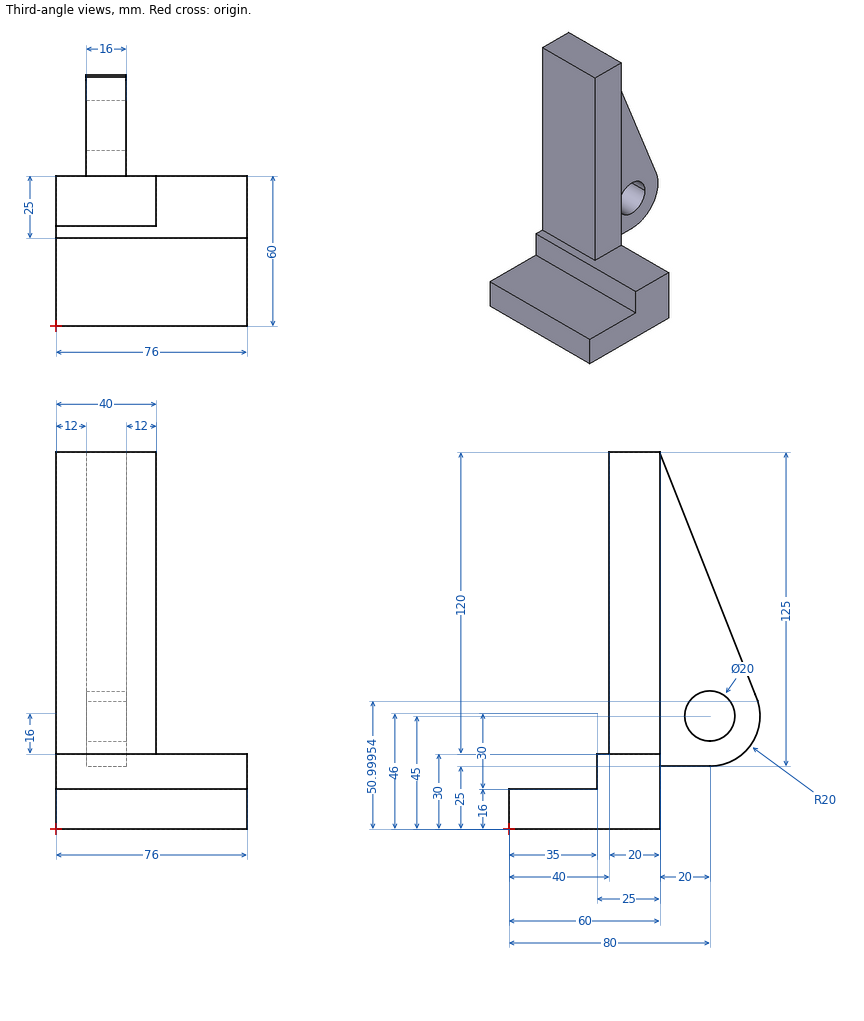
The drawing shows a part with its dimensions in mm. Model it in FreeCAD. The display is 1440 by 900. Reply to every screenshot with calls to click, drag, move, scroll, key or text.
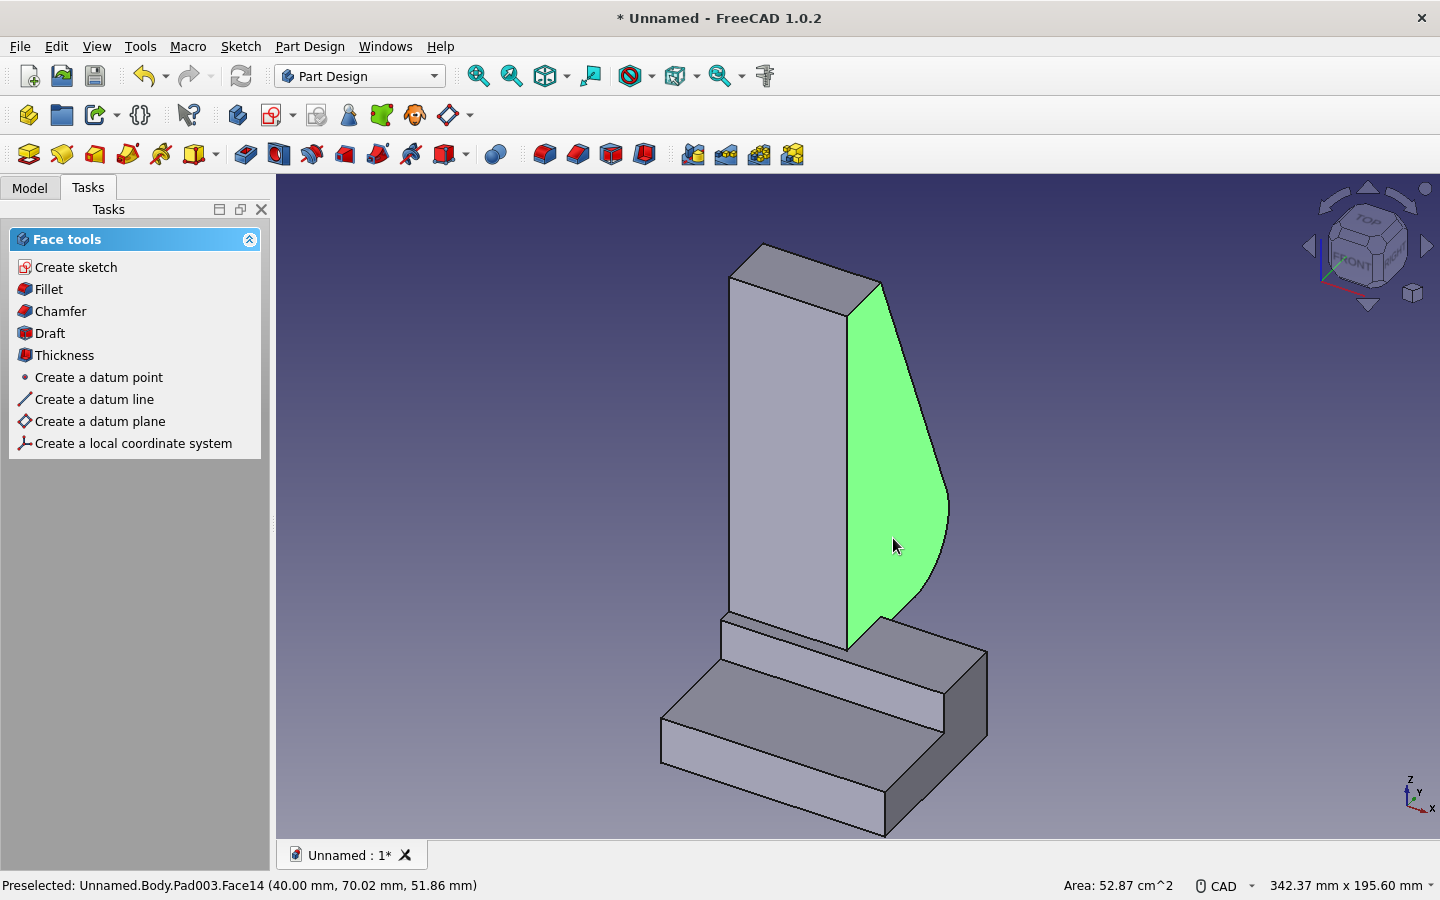
click(270, 116)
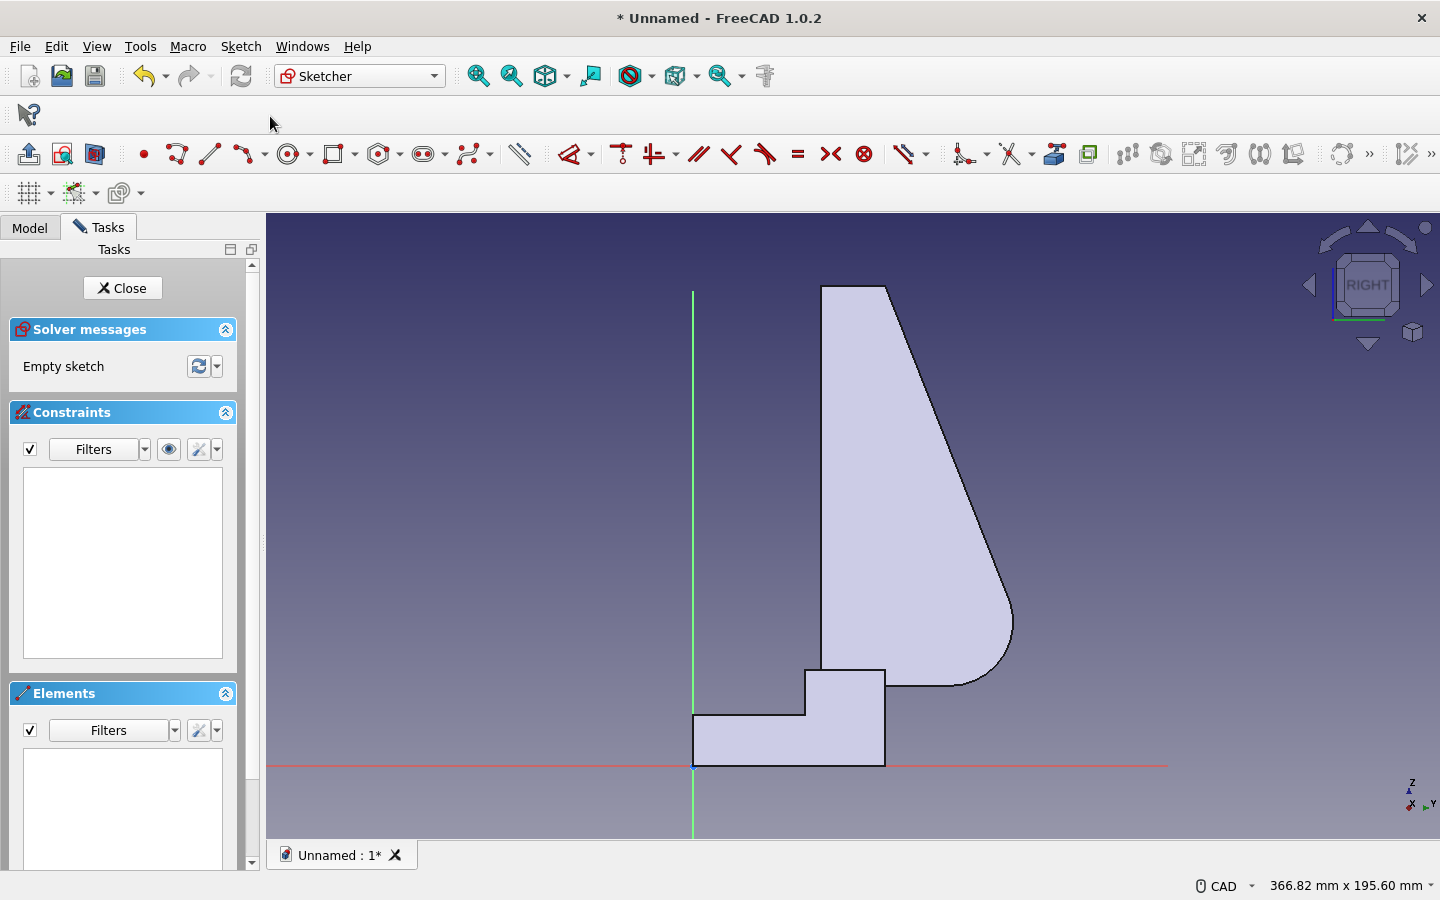
key(g)
key(m)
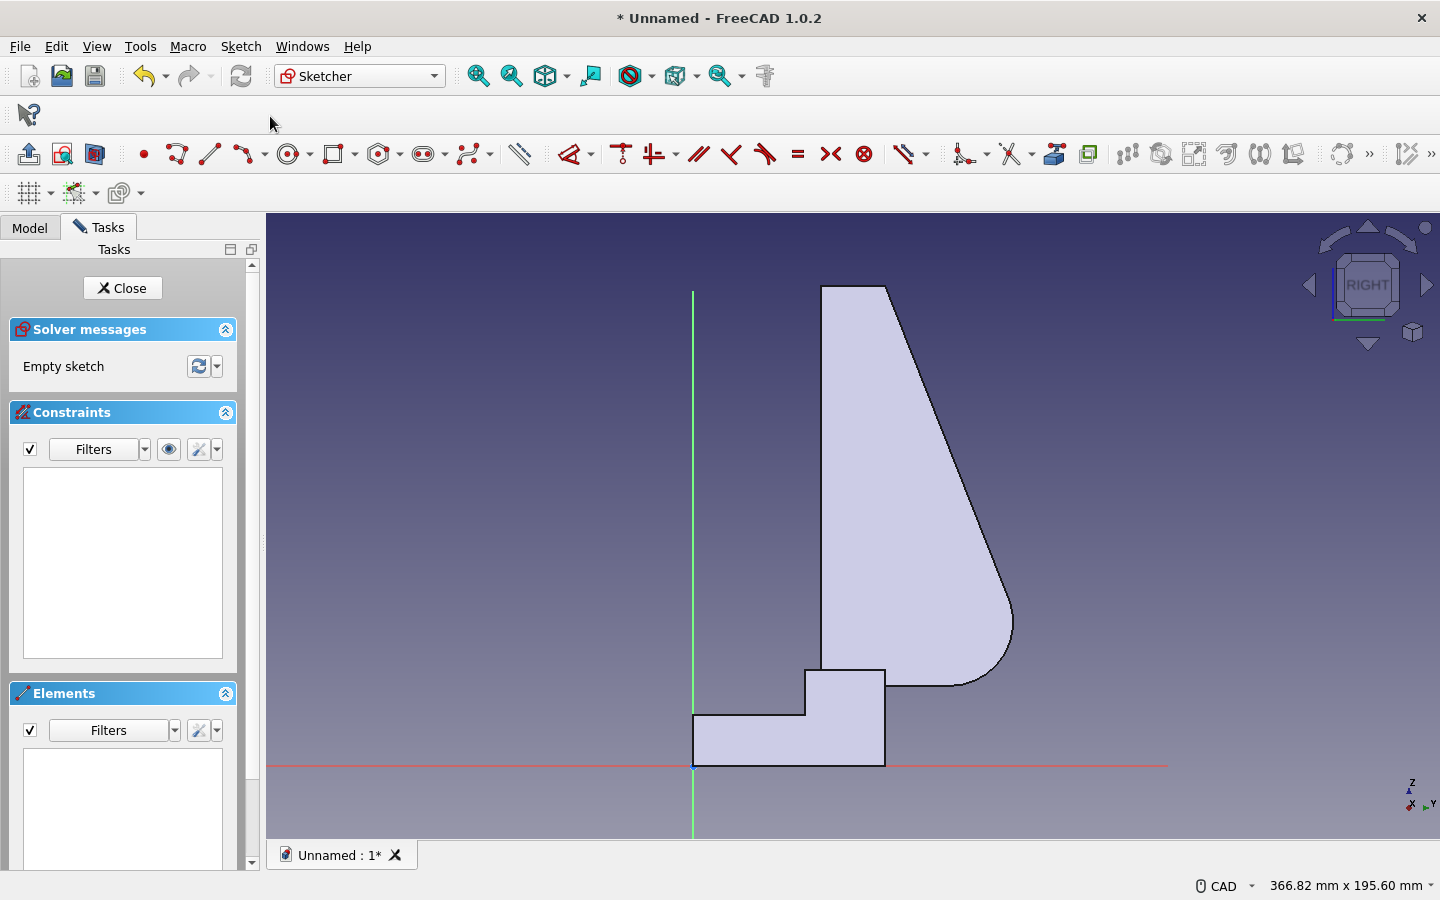
click(1010, 603)
click(885, 286)
click(885, 686)
click(949, 686)
right_click(949, 686)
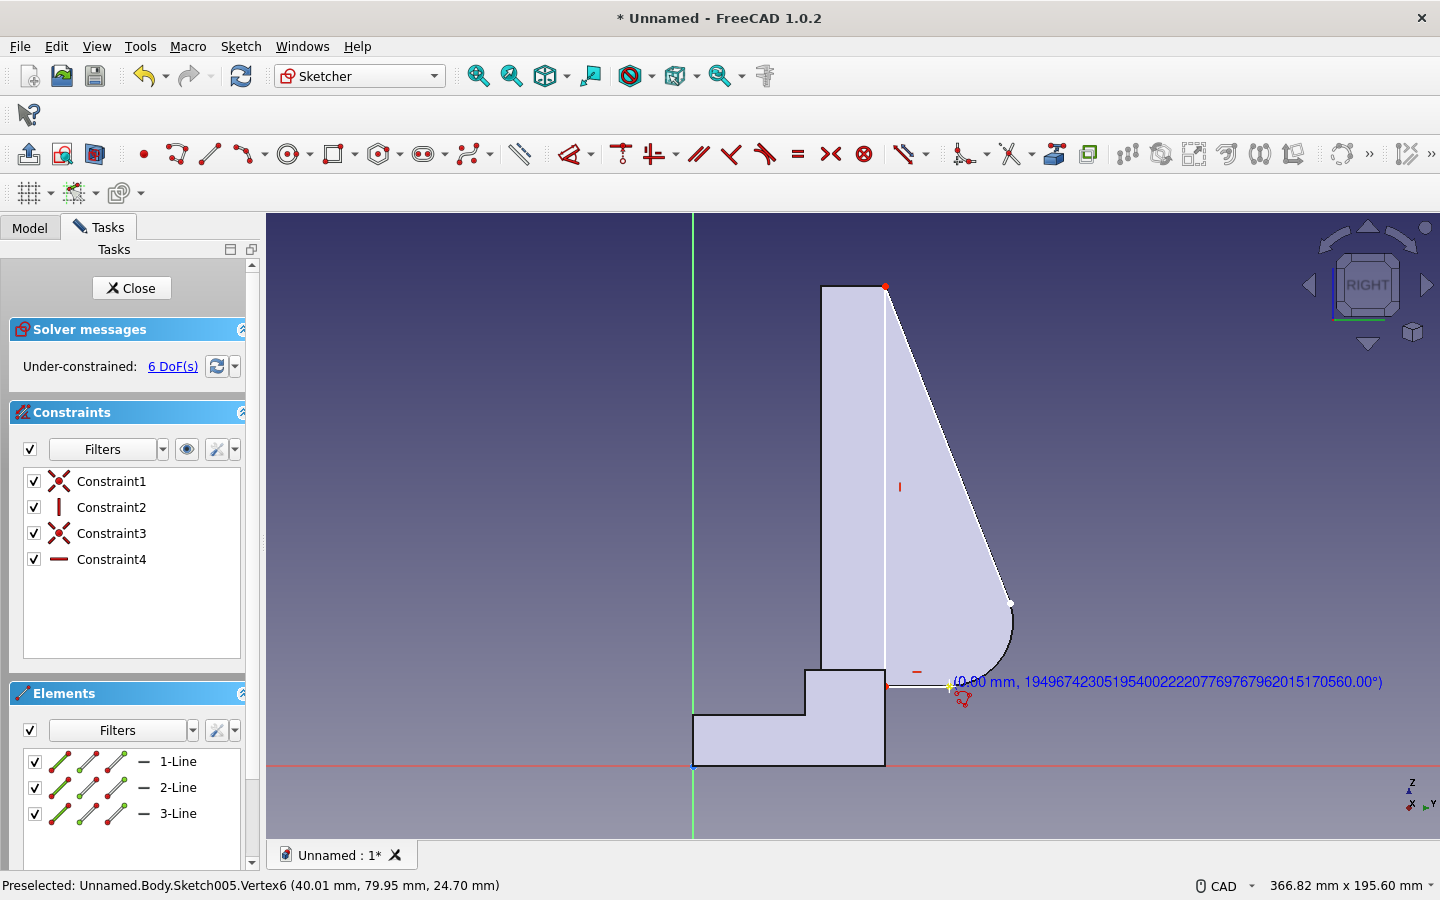
key(g)
key(3)
key(a)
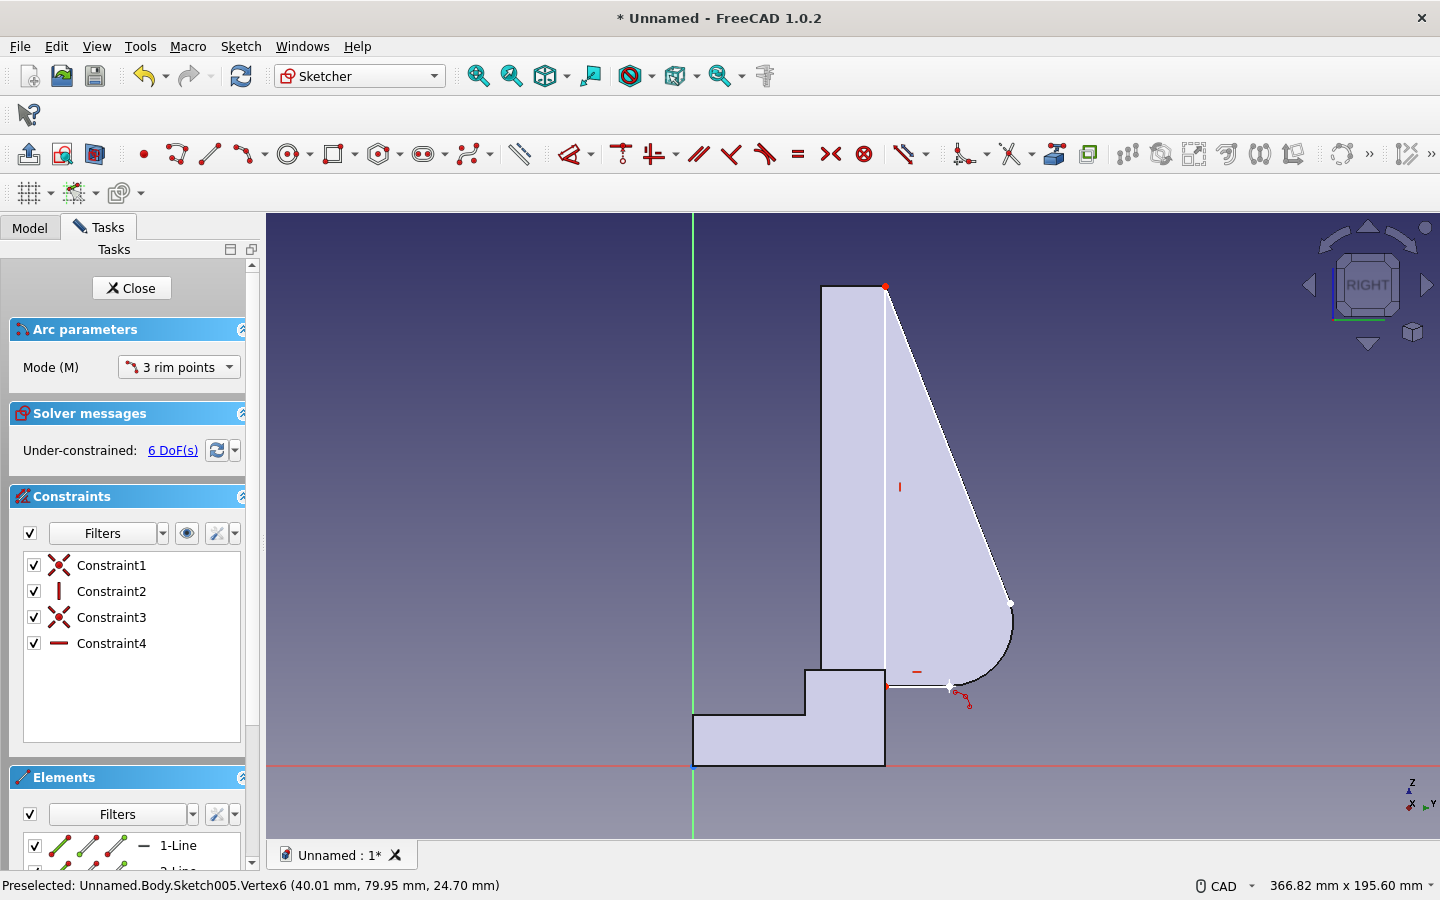
click(949, 687)
click(1010, 604)
click(1001, 660)
key(Escape)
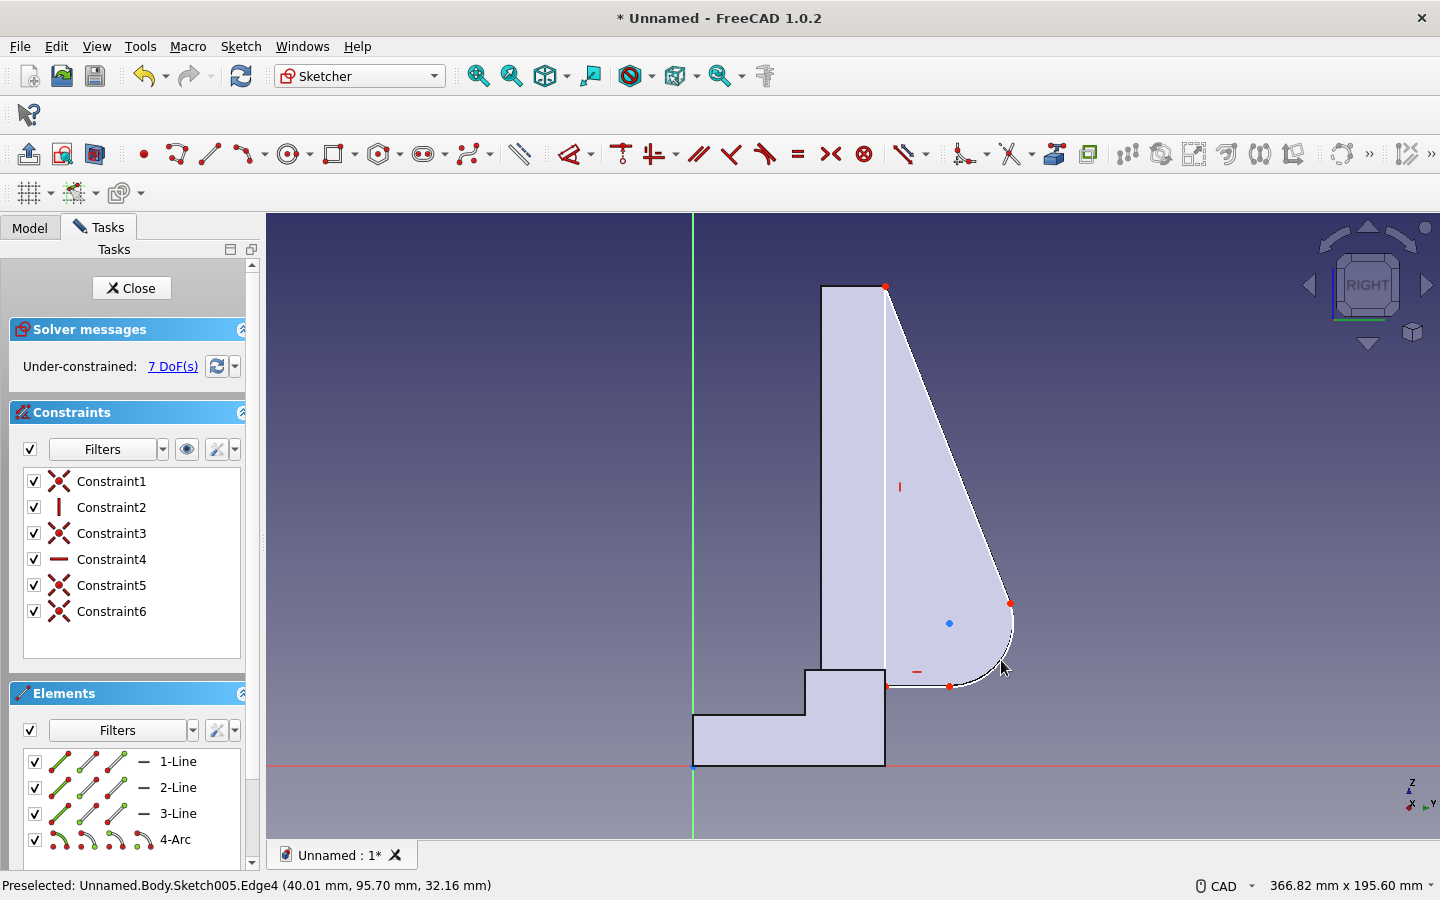
click(904, 687)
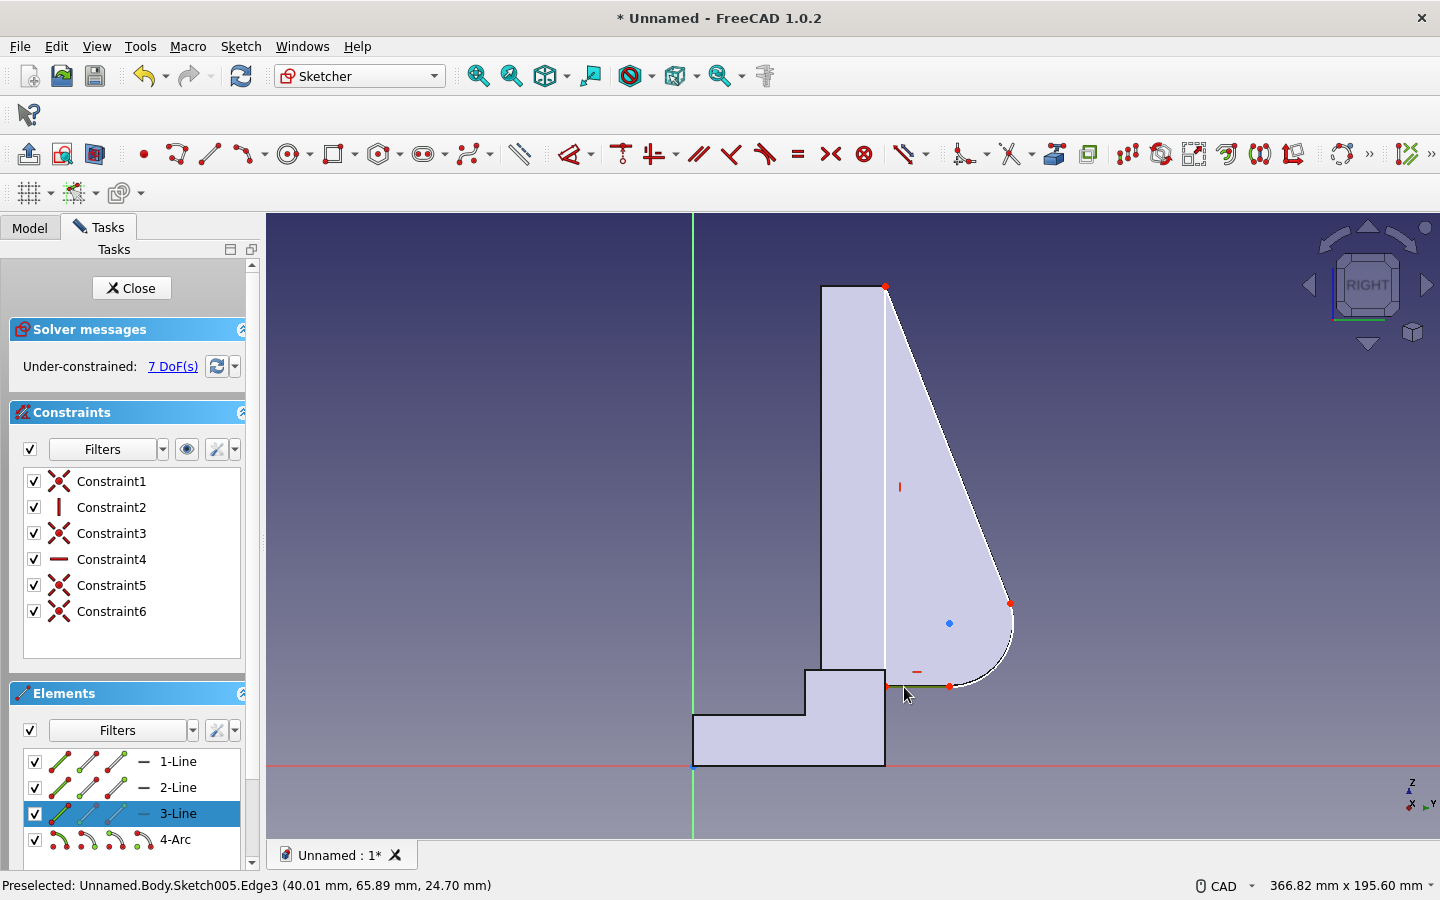
click(983, 677)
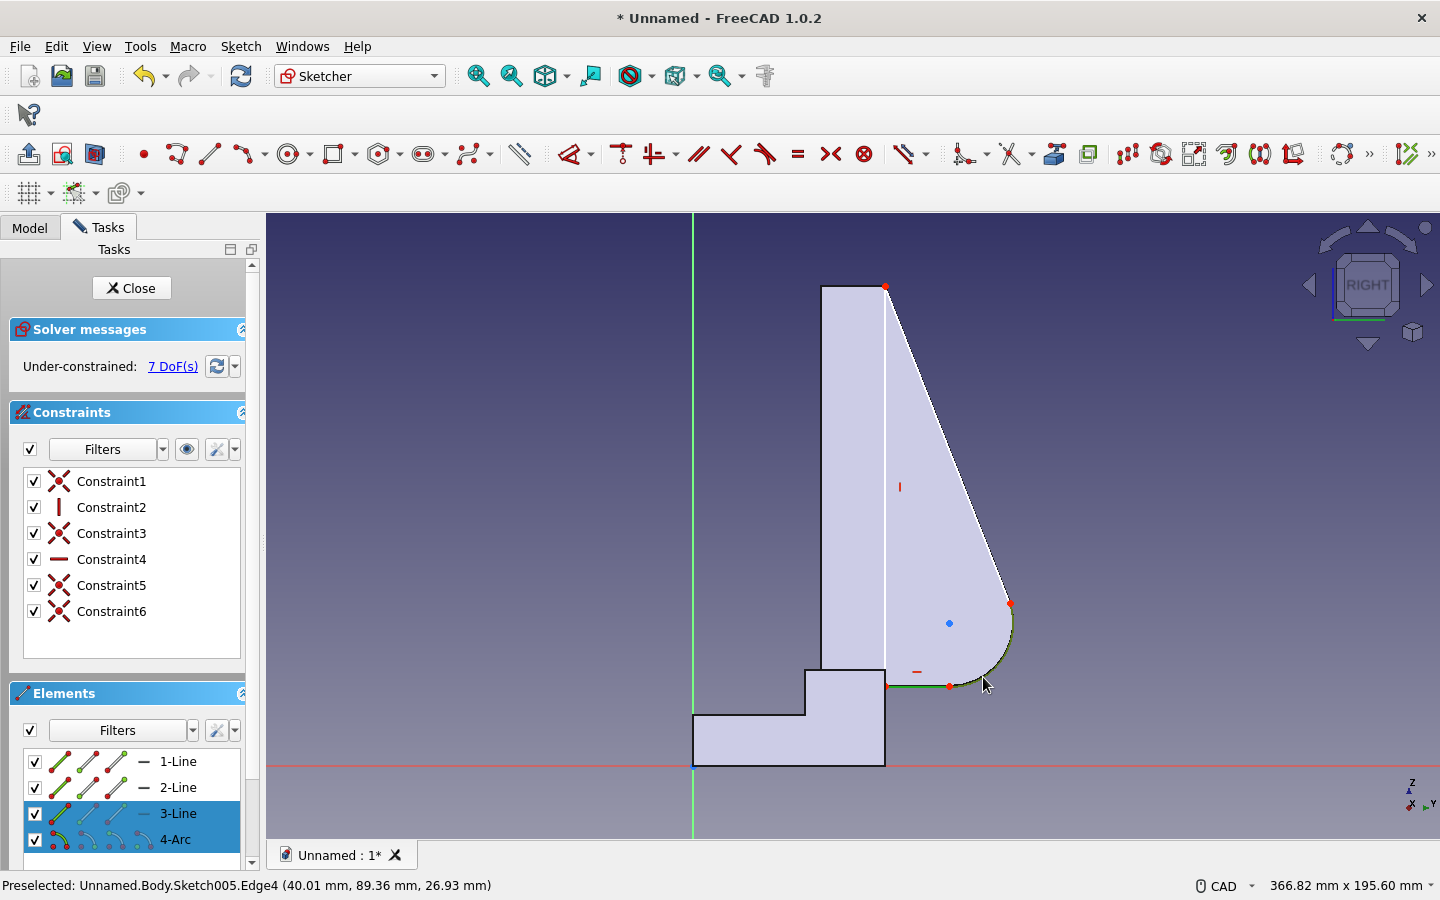
key(t)